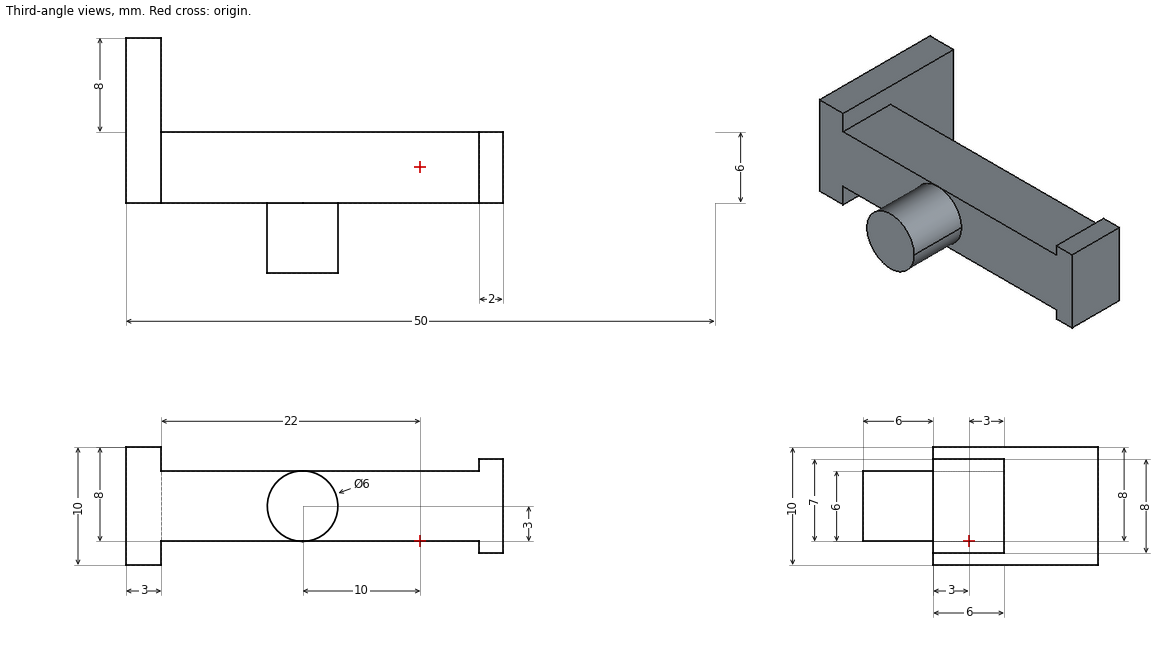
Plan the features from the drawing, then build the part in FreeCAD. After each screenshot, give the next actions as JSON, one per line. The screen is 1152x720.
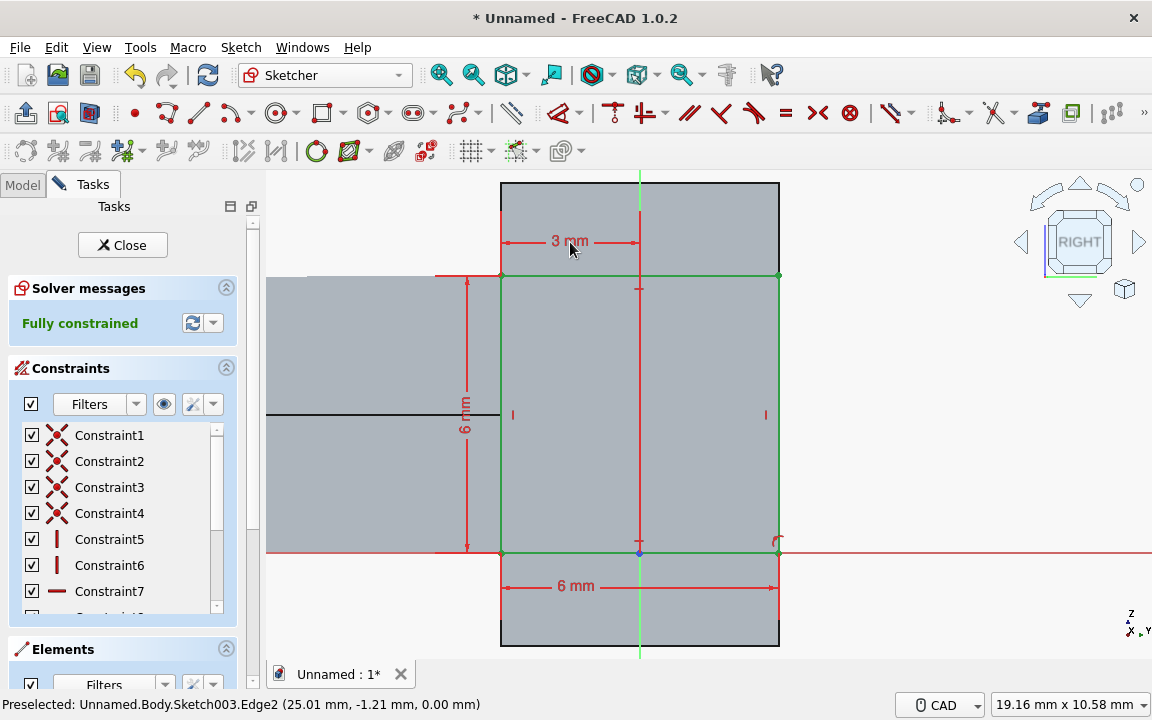
{"action": "left_click", "coordinate": [123, 245]}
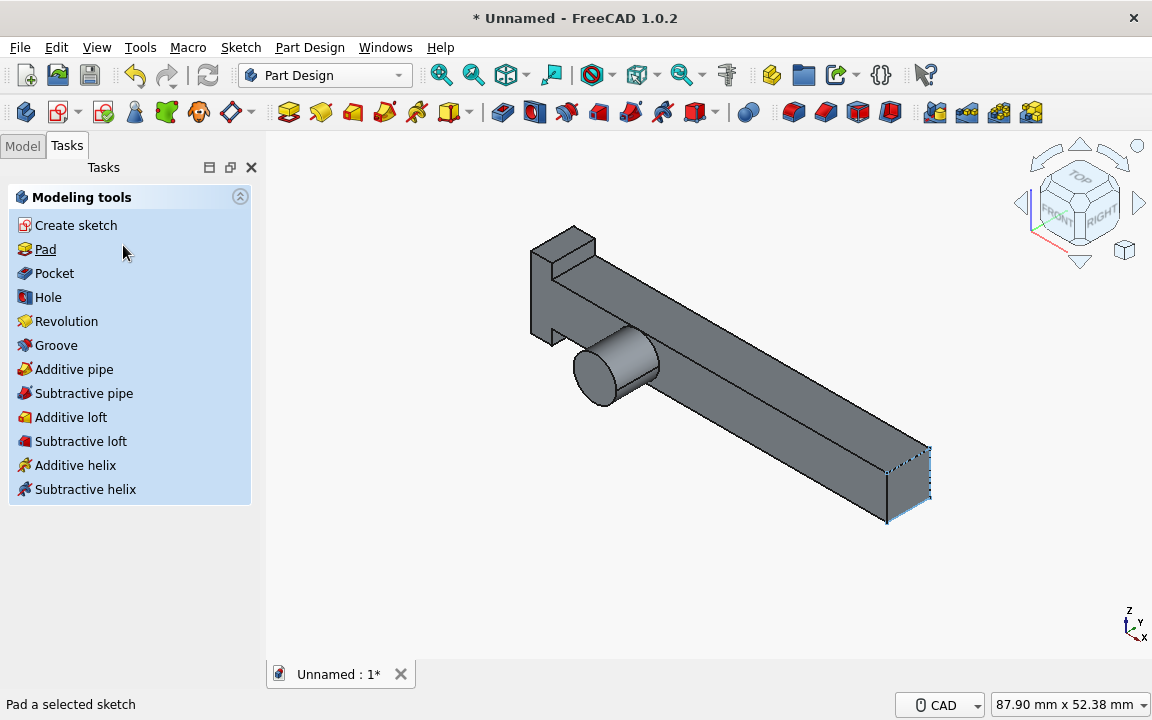
{"action": "left_click", "coordinate": [504, 112]}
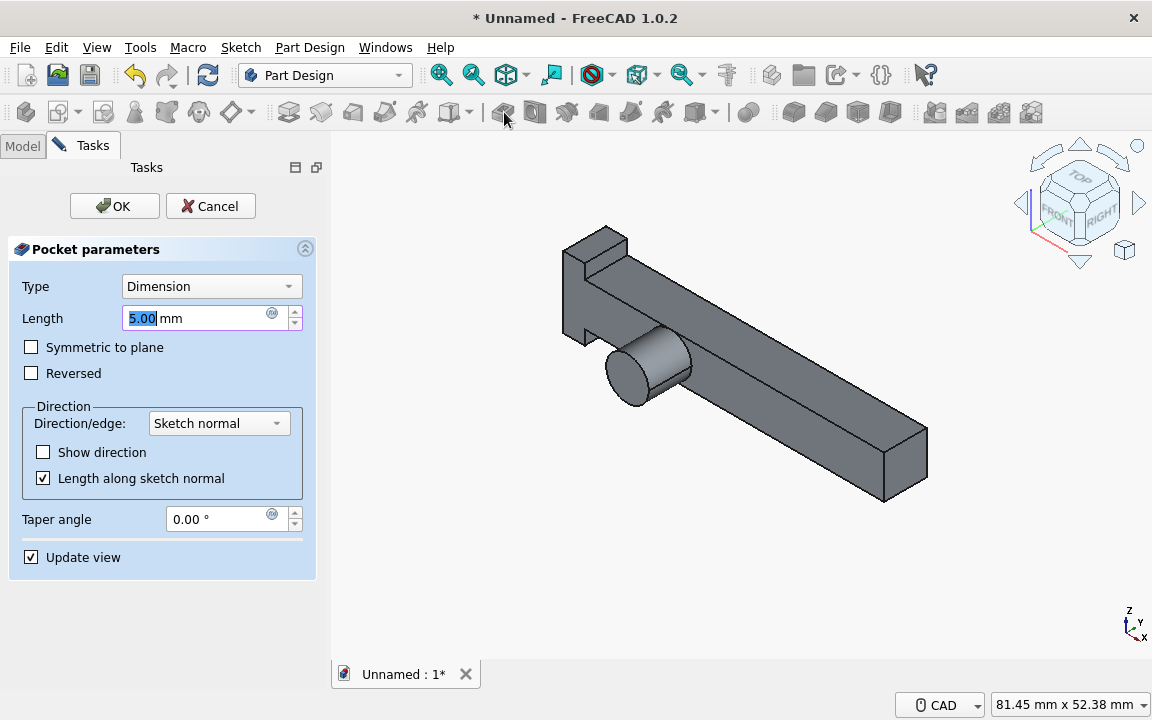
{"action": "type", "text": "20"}
{"action": "key", "text": "Tab"}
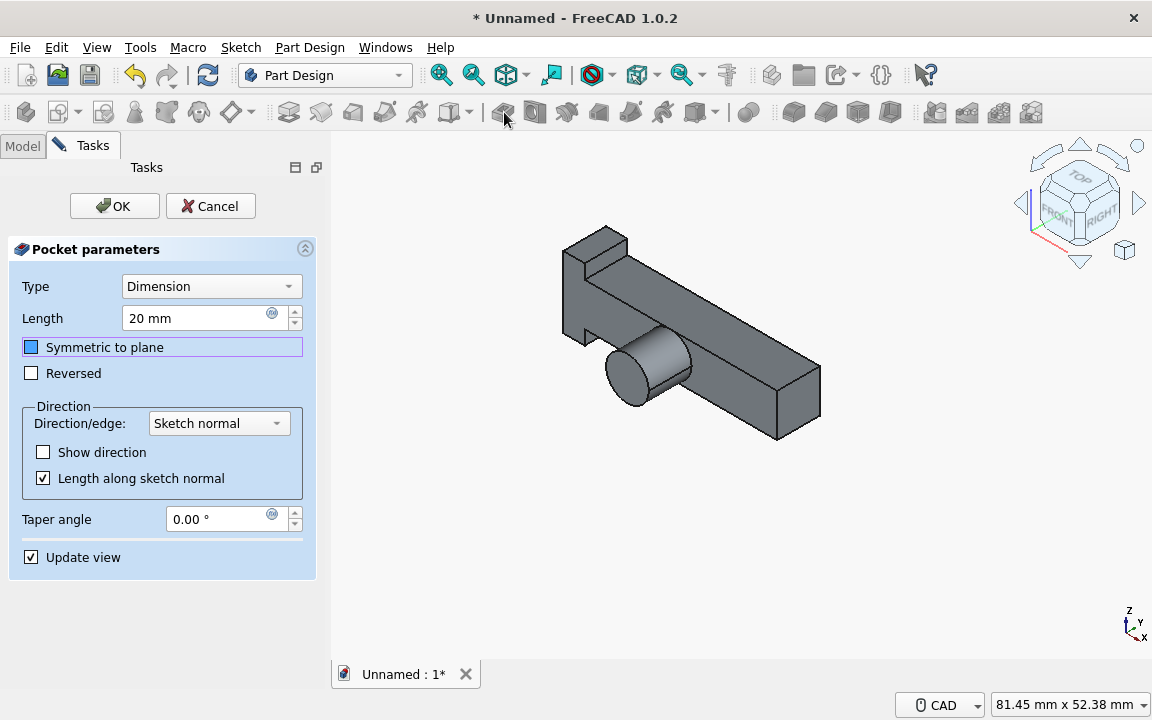
{"action": "left_click", "coordinate": [115, 206]}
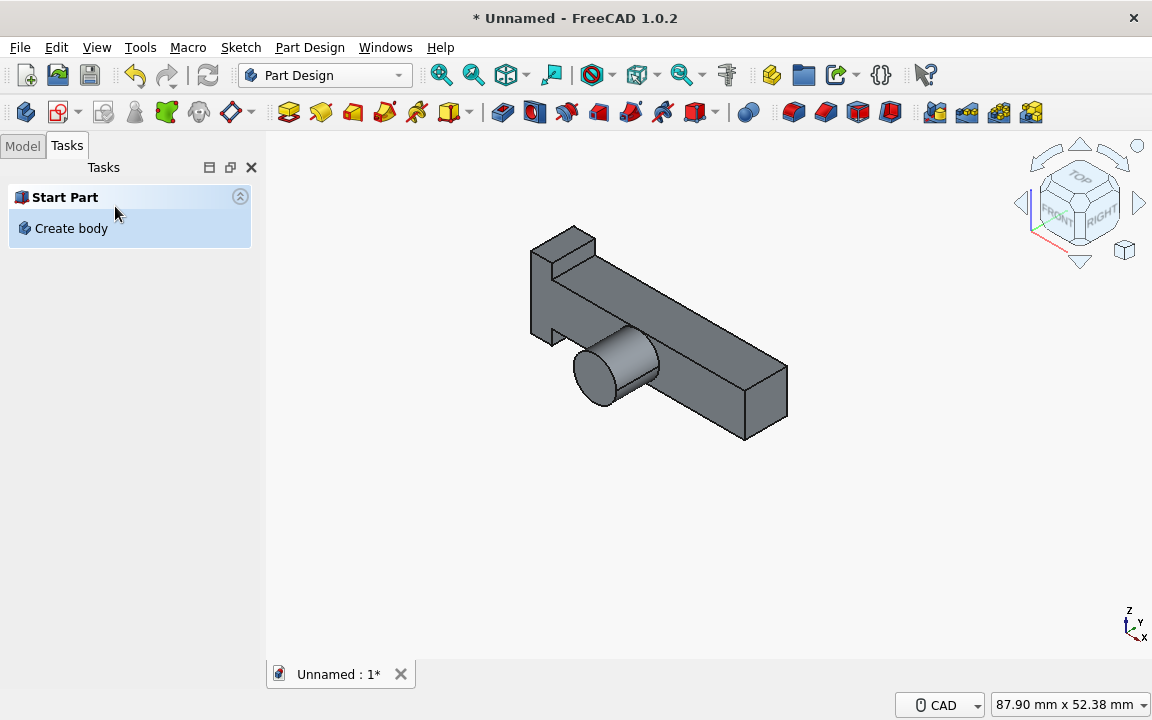
{"action": "left_click", "coordinate": [766, 402]}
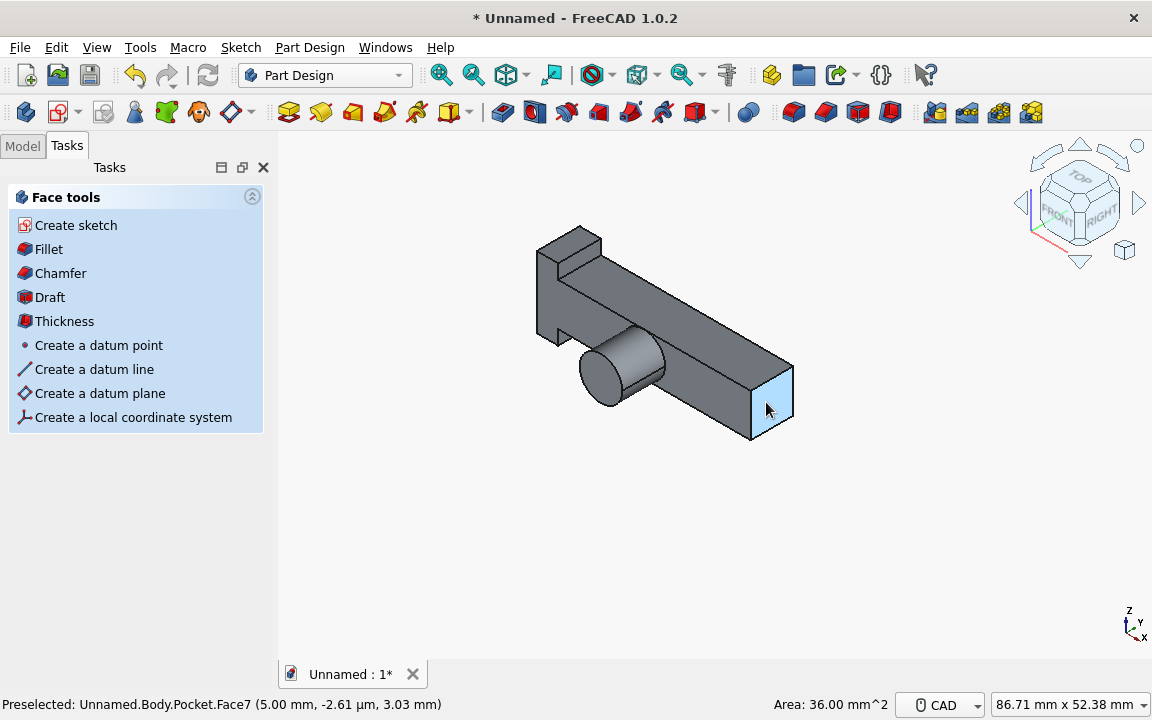
{"action": "left_click", "coordinate": [58, 112]}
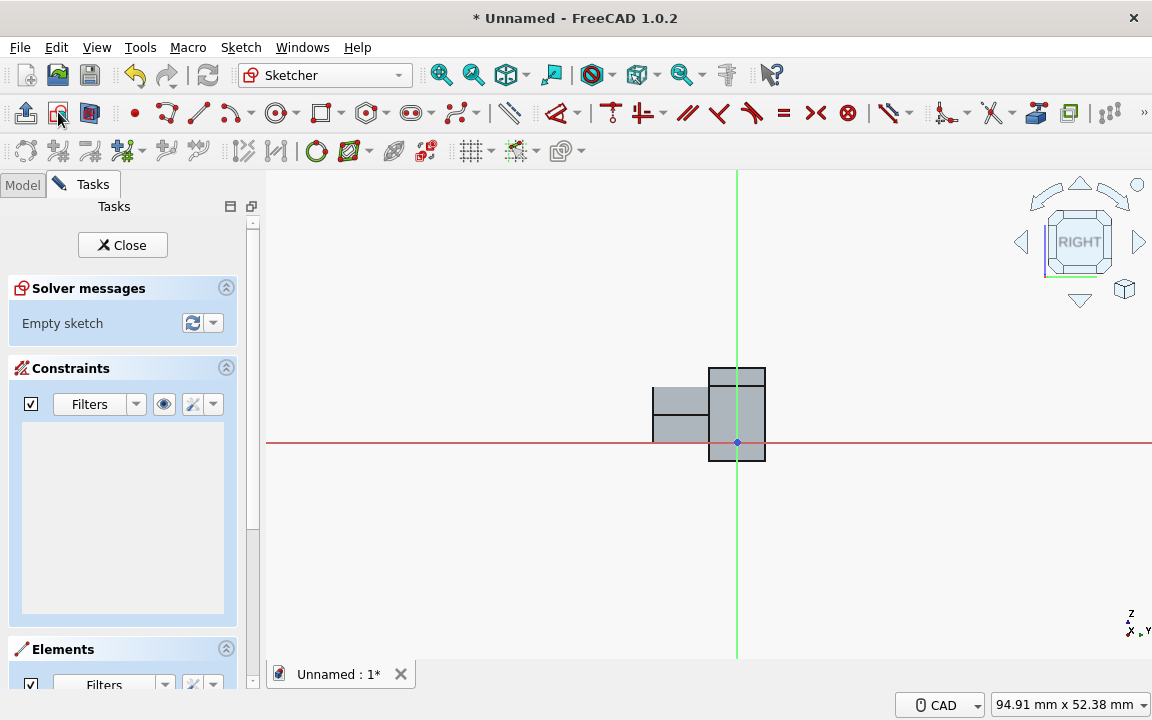
{"action": "scroll", "coordinate": [769, 414], "scroll_direction": "up", "scroll_amount": 7}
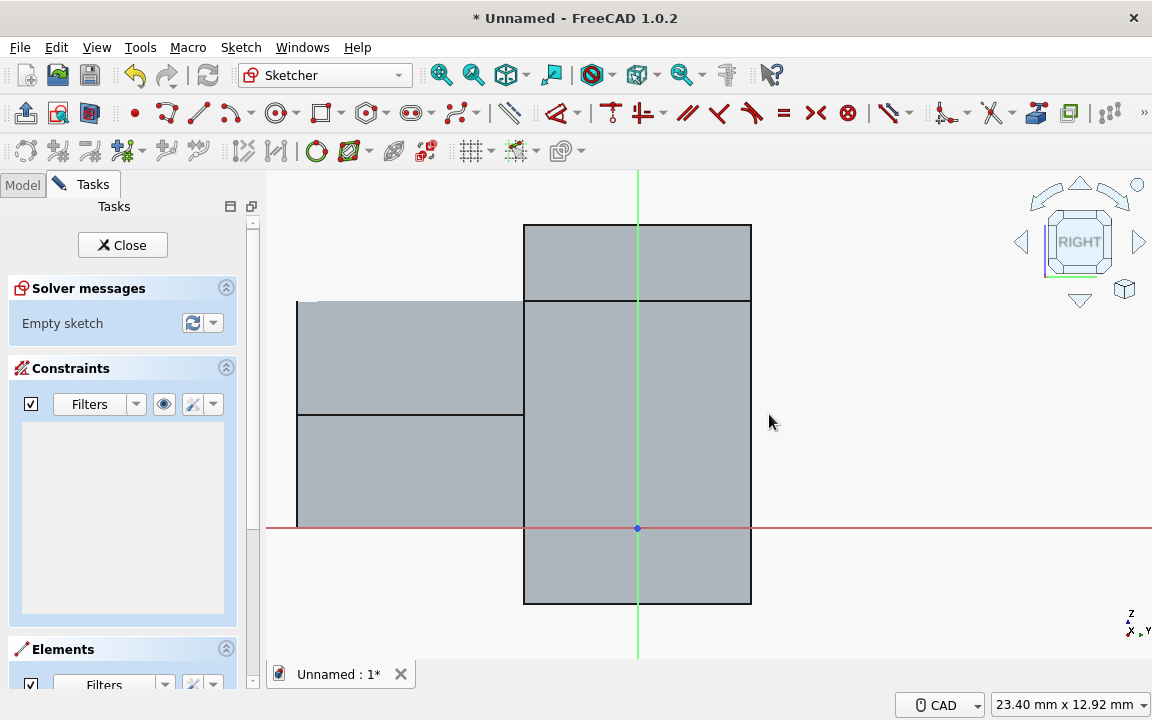
{"action": "left_click", "coordinate": [322, 114]}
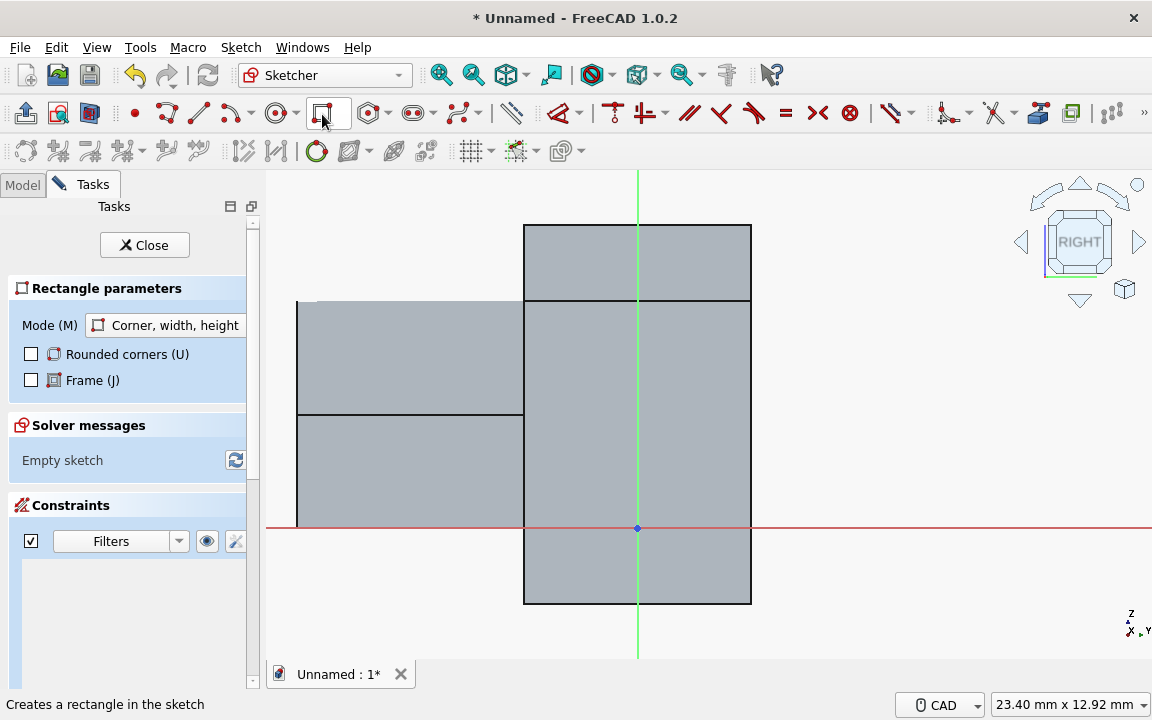
{"action": "left_click", "coordinate": [524, 263]}
{"action": "mouse_move", "coordinate": [751, 566]}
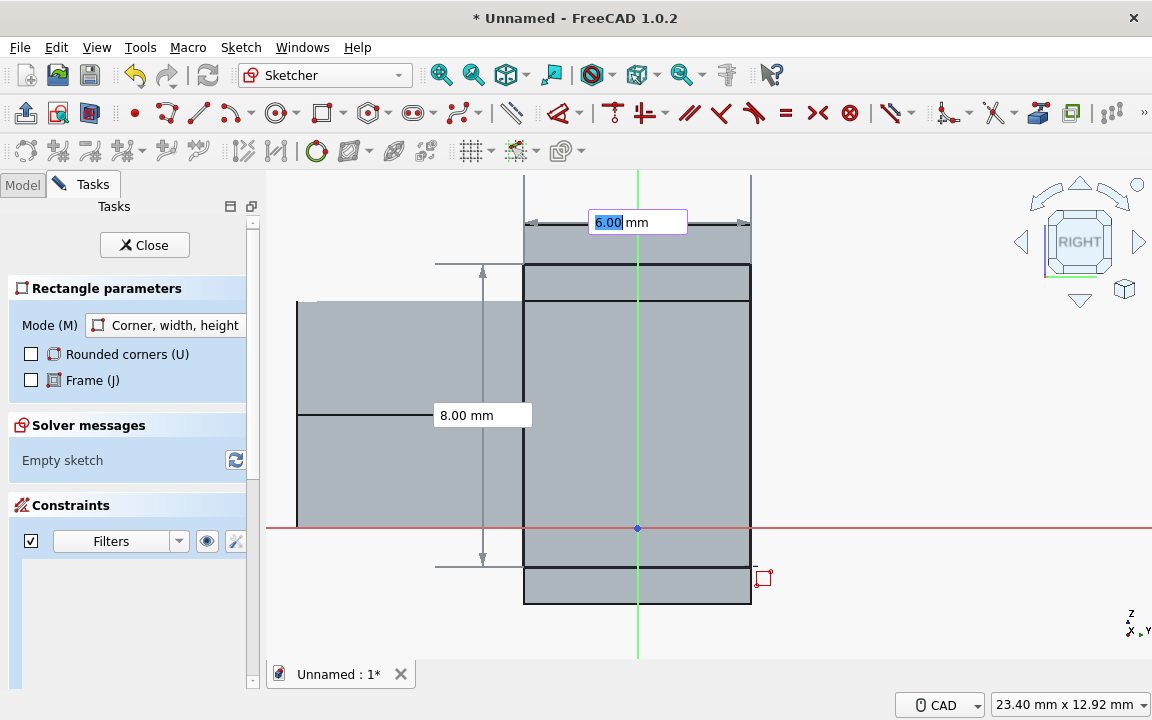
{"action": "type", "text": "6"}
{"action": "key", "text": "Tab"}
{"action": "type", "text": "8"}
{"action": "key", "text": "Return"}
{"action": "key", "text": "Escape"}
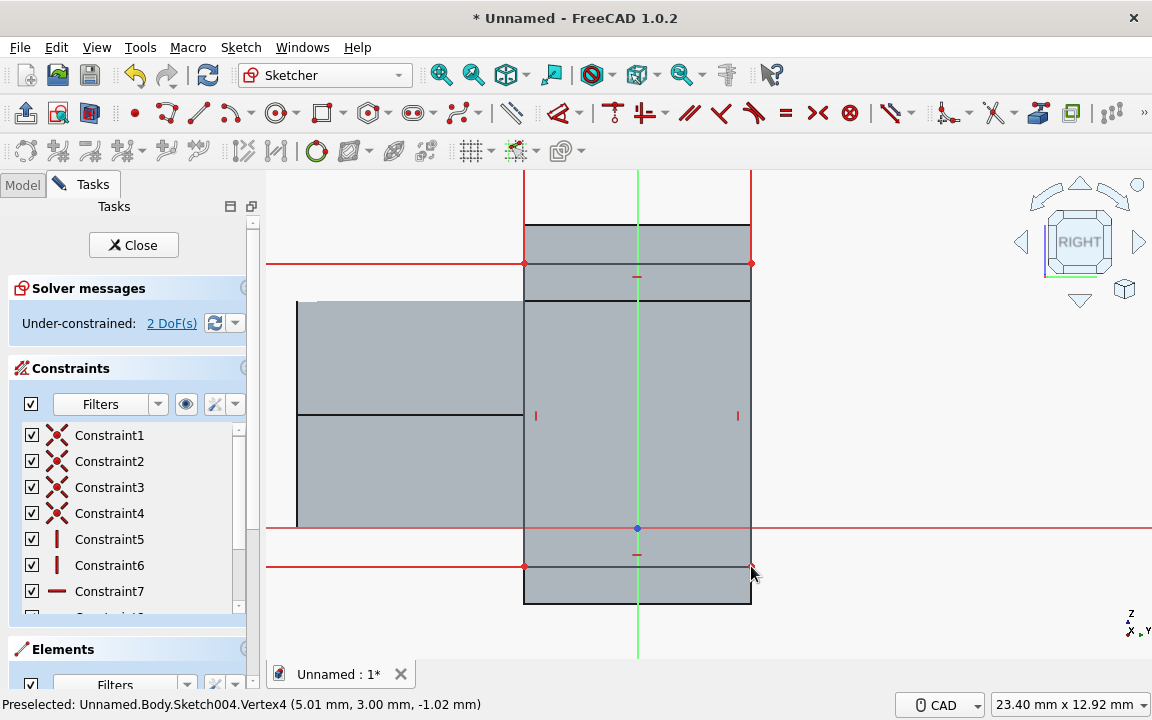
{"action": "left_click", "coordinate": [558, 114]}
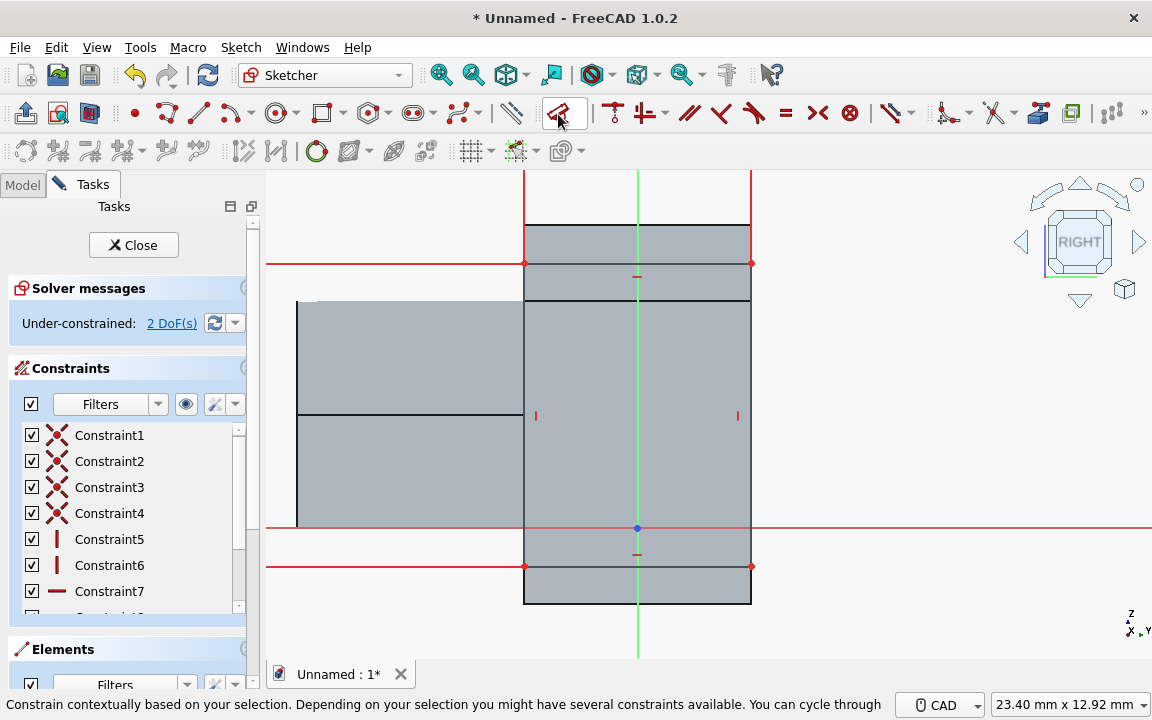
{"action": "left_click", "coordinate": [524, 264]}
{"action": "left_click", "coordinate": [581, 230]}